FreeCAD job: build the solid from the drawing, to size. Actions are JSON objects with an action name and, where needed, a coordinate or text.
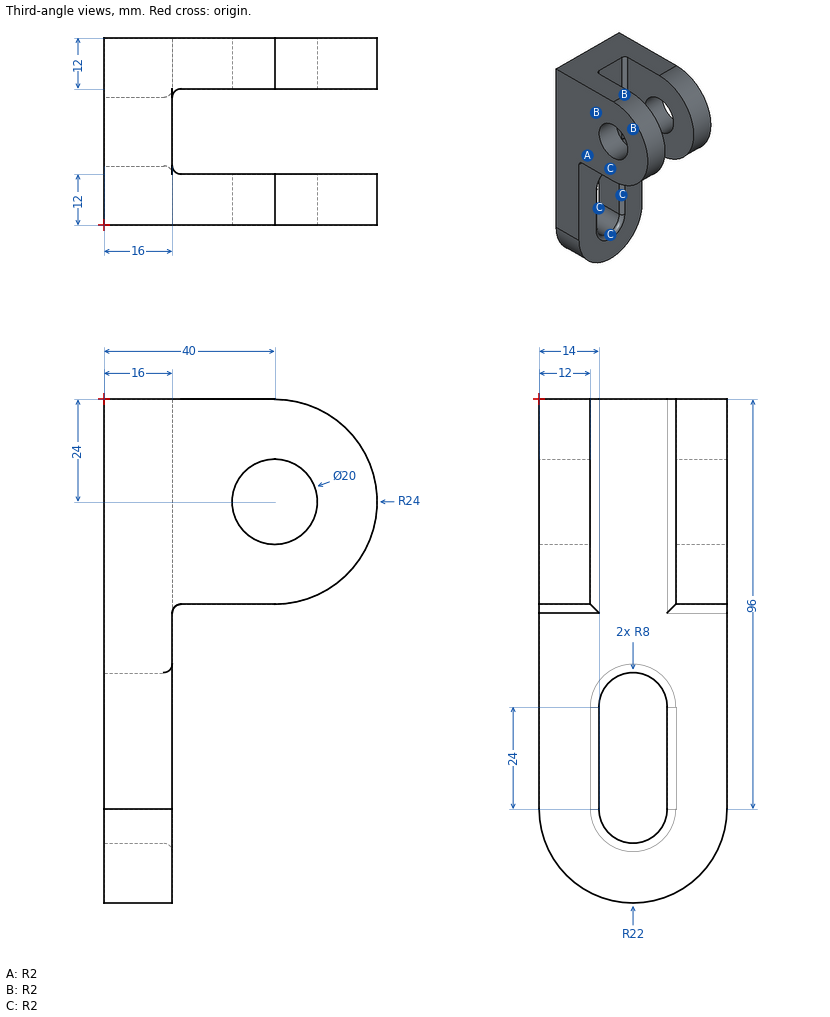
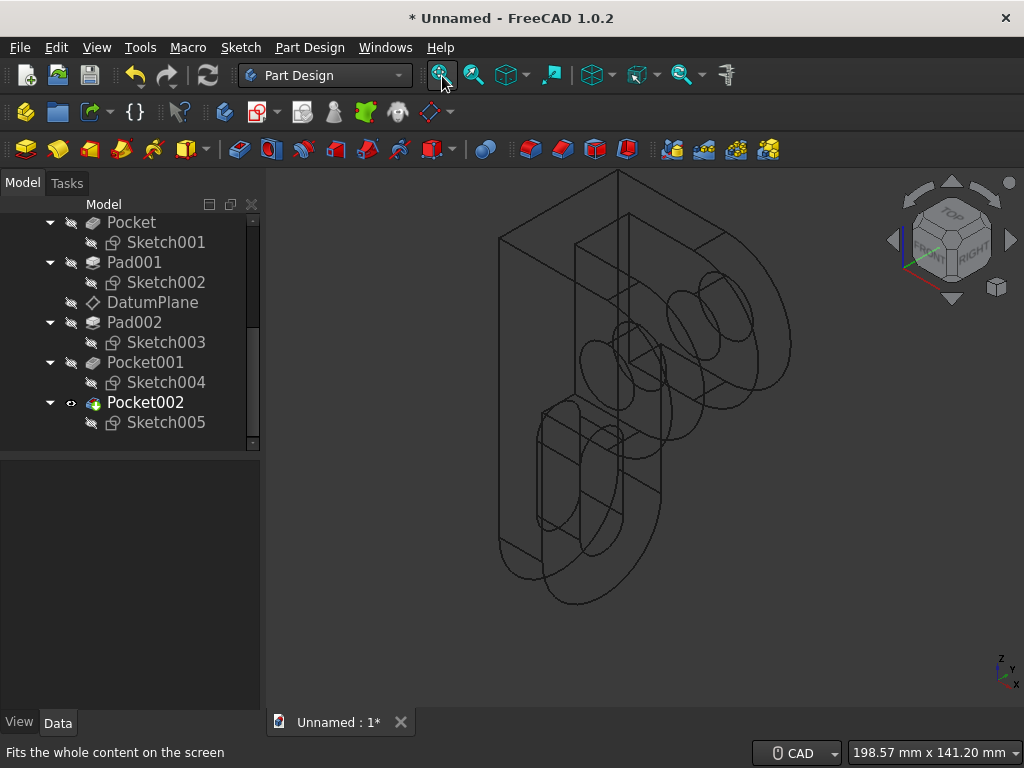
{"action": "left_click", "coordinate": [559, 402]}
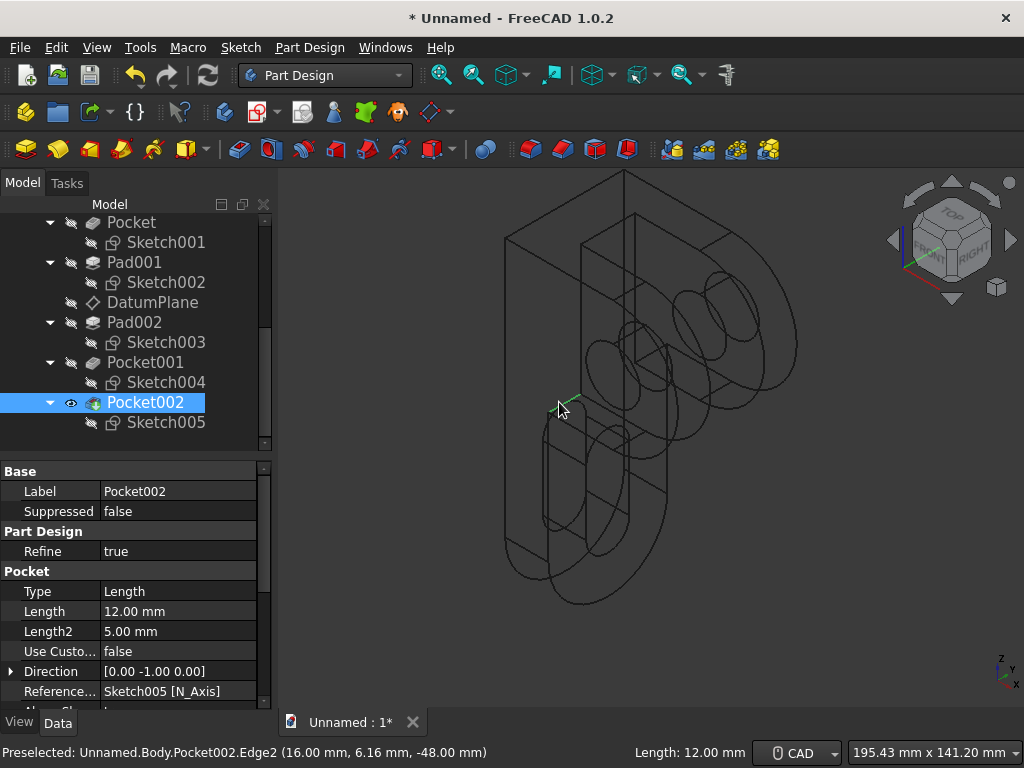
{"action": "key", "text": "v 1"}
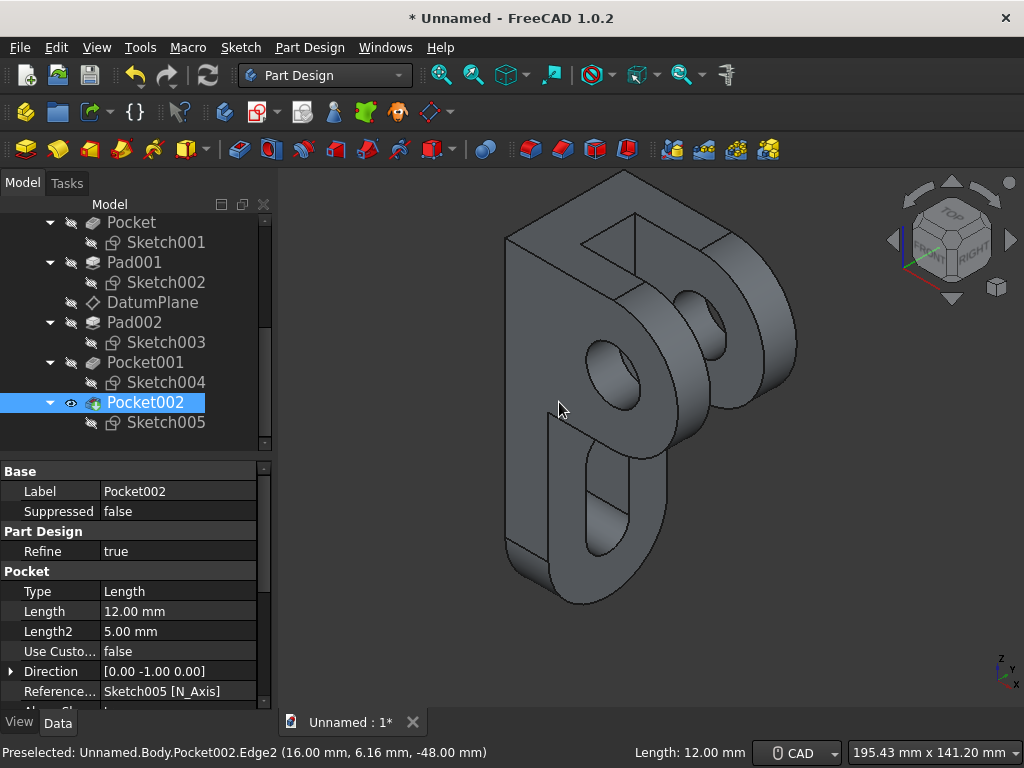
{"action": "left_click", "coordinate": [532, 150]}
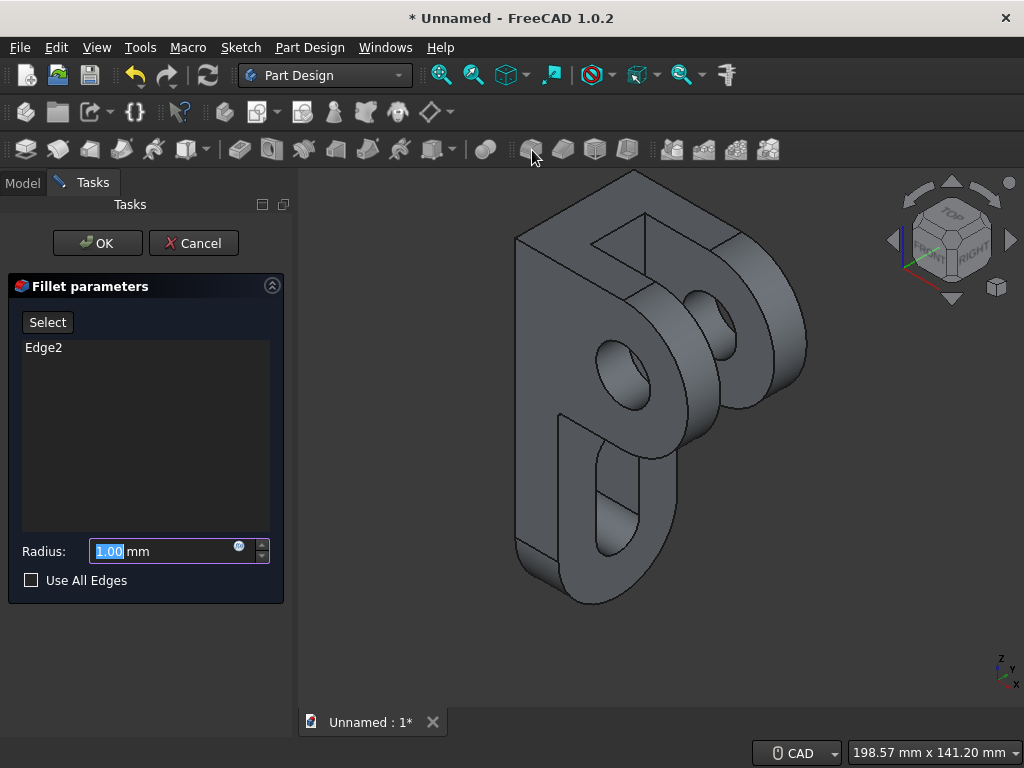
{"action": "type", "text": "2"}
{"action": "key", "text": "Tab"}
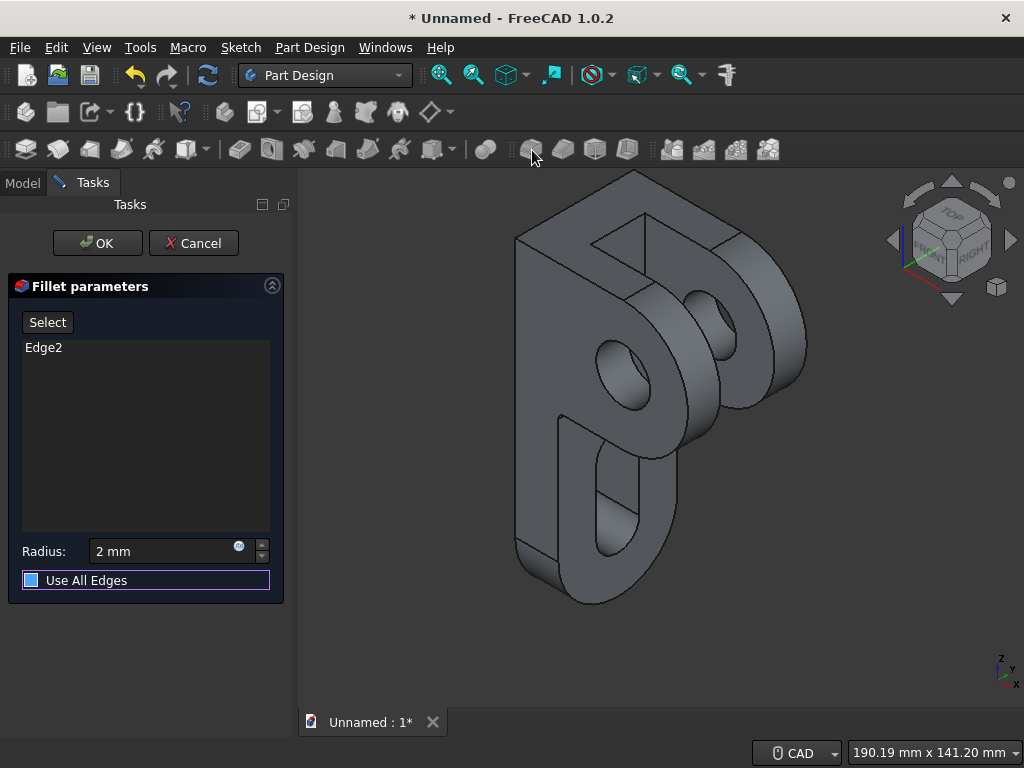
{"action": "left_click", "coordinate": [98, 243]}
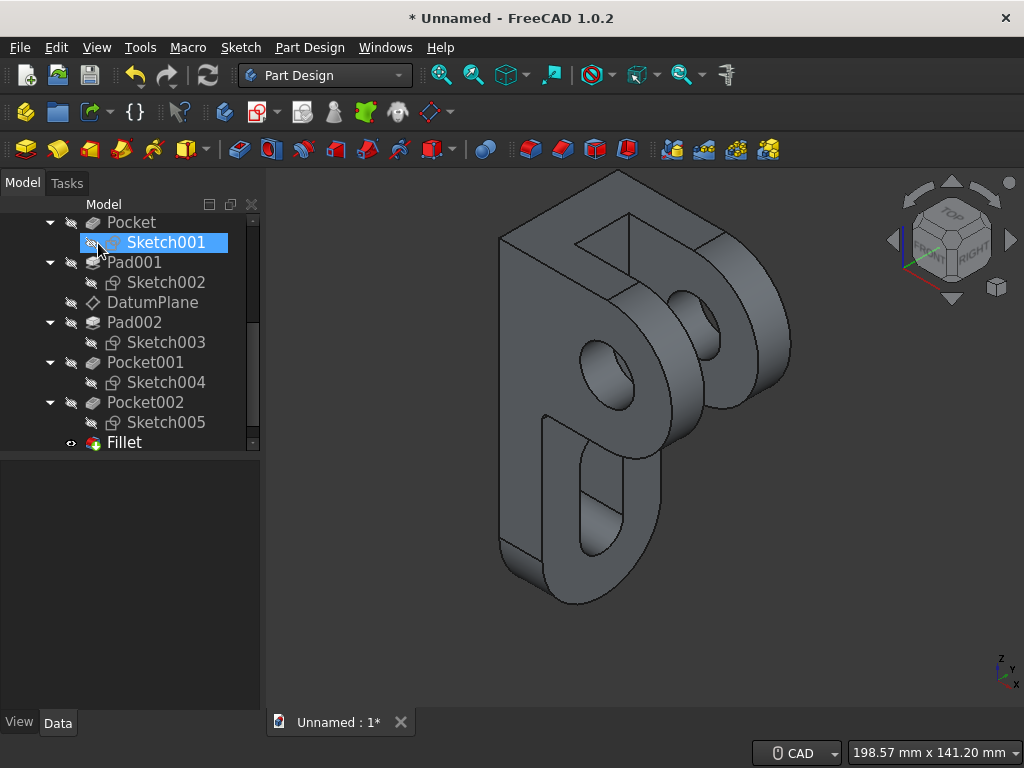
{"action": "key", "text": "2"}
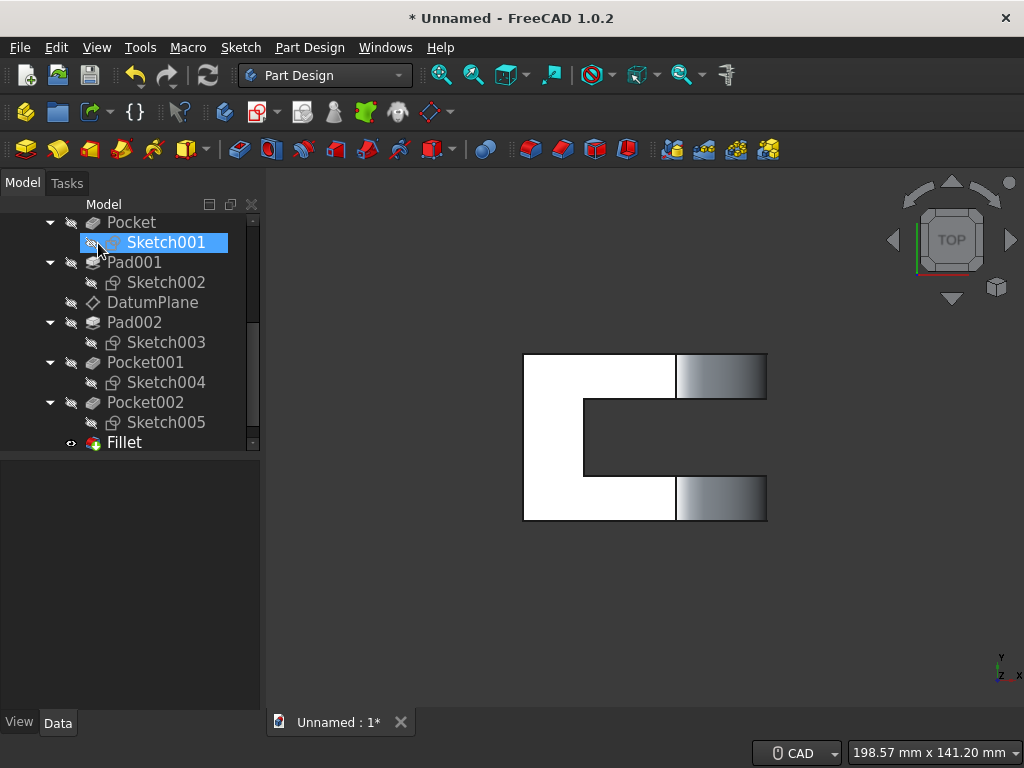
{"action": "left_click", "coordinate": [442, 76]}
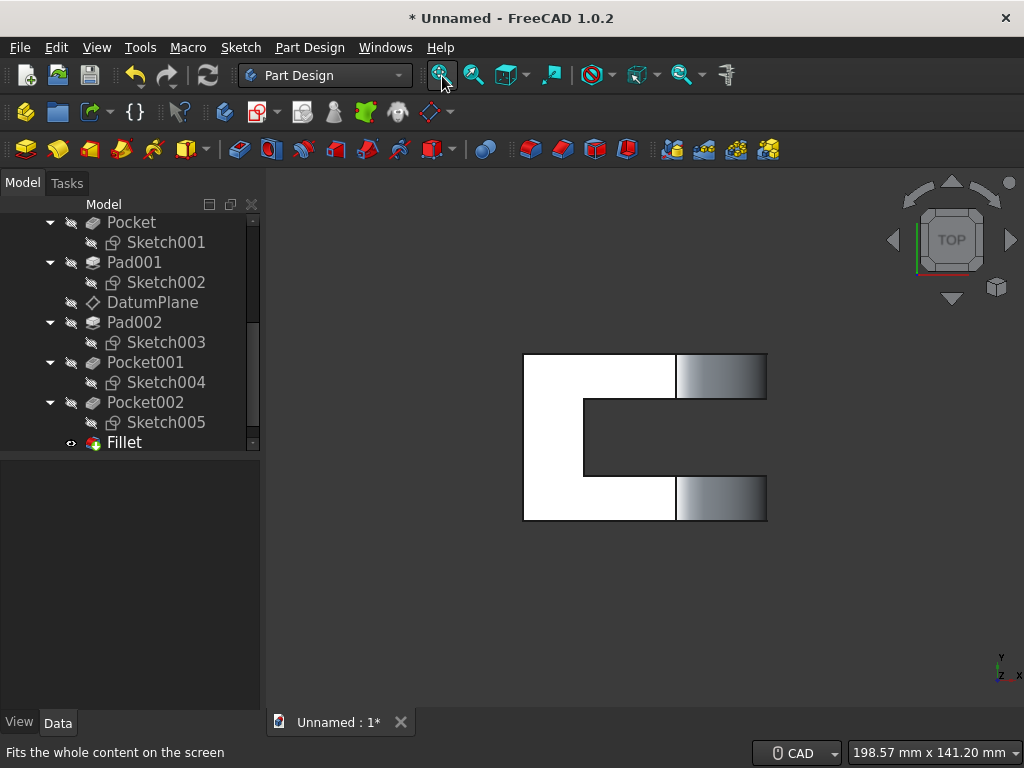
{"action": "key", "text": "0"}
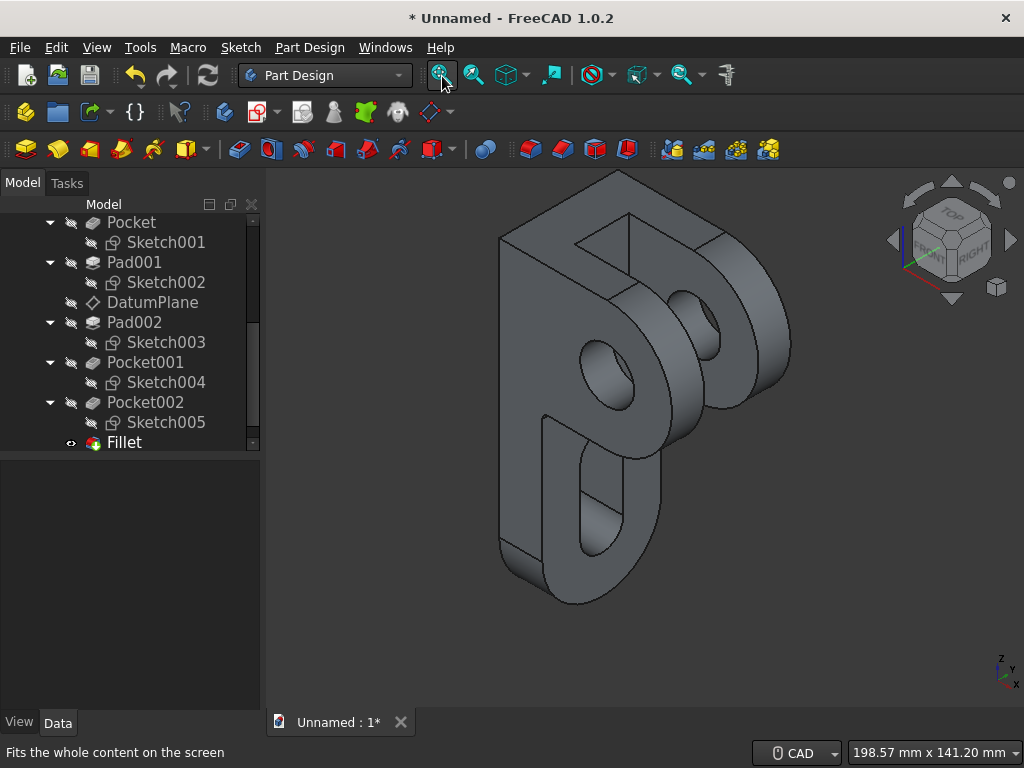
{"action": "key", "text": "1"}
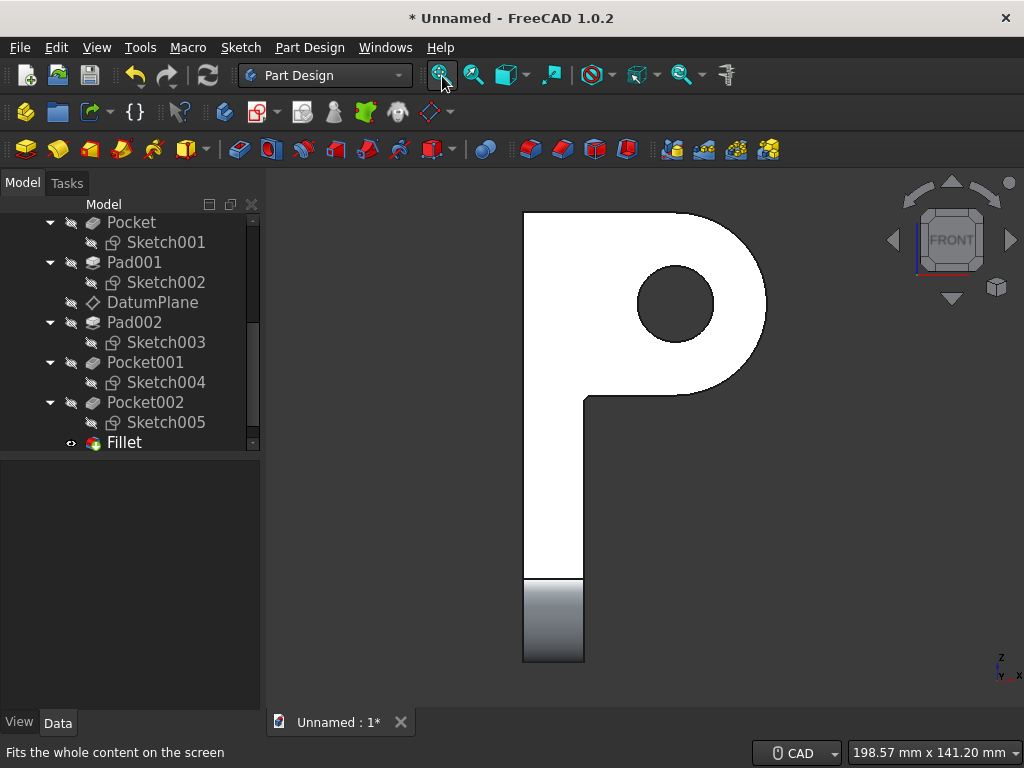
{"action": "key", "text": "3"}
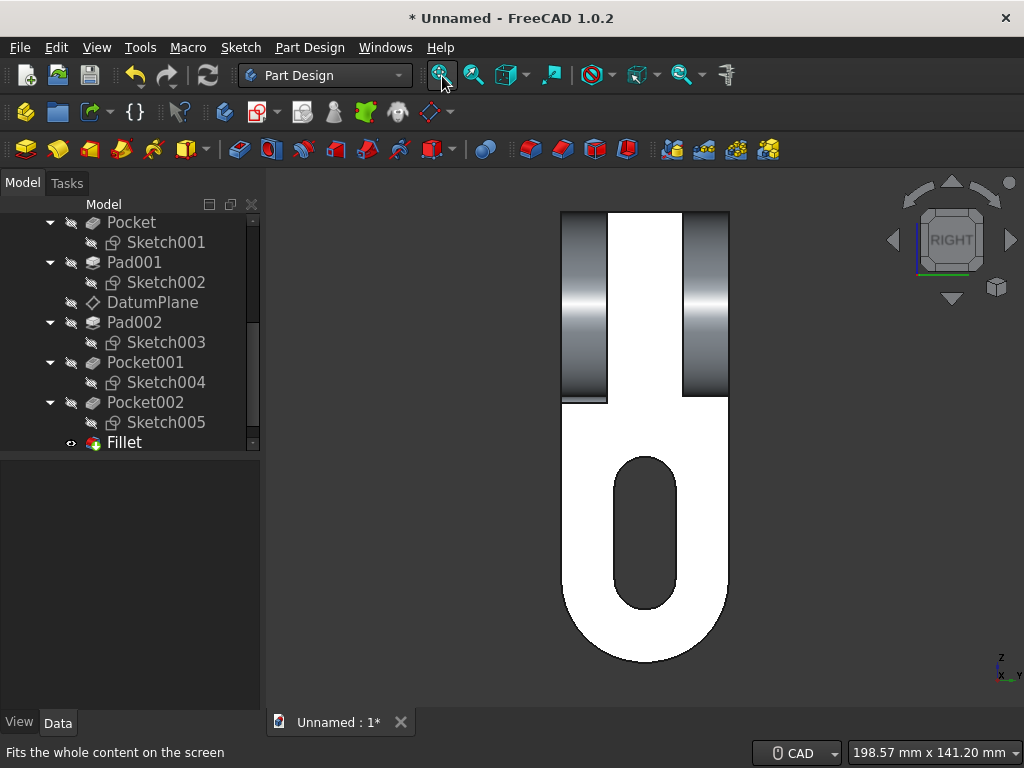
{"action": "key", "text": "5"}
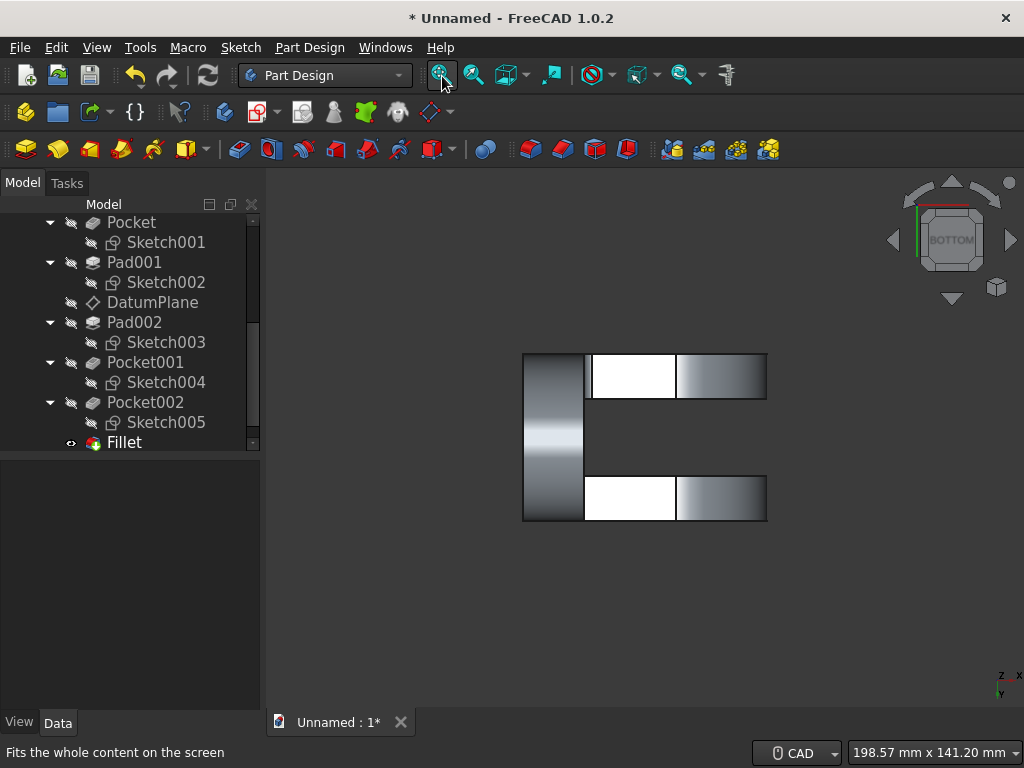
{"action": "left_click", "coordinate": [442, 76]}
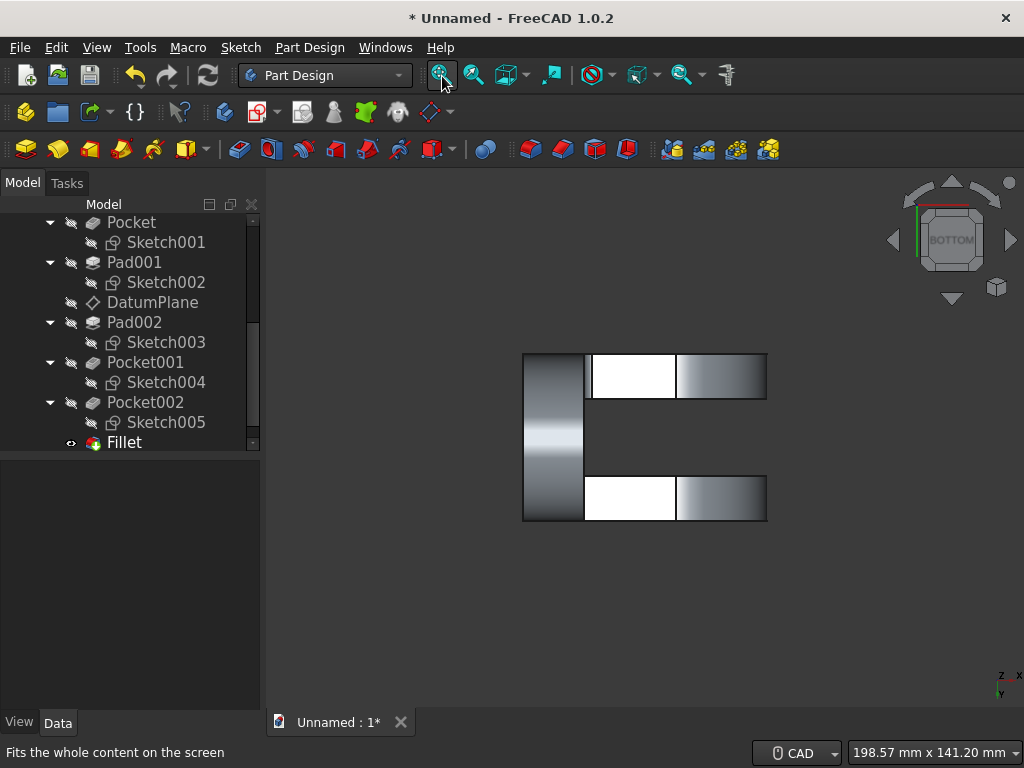
{"action": "key", "text": "4"}